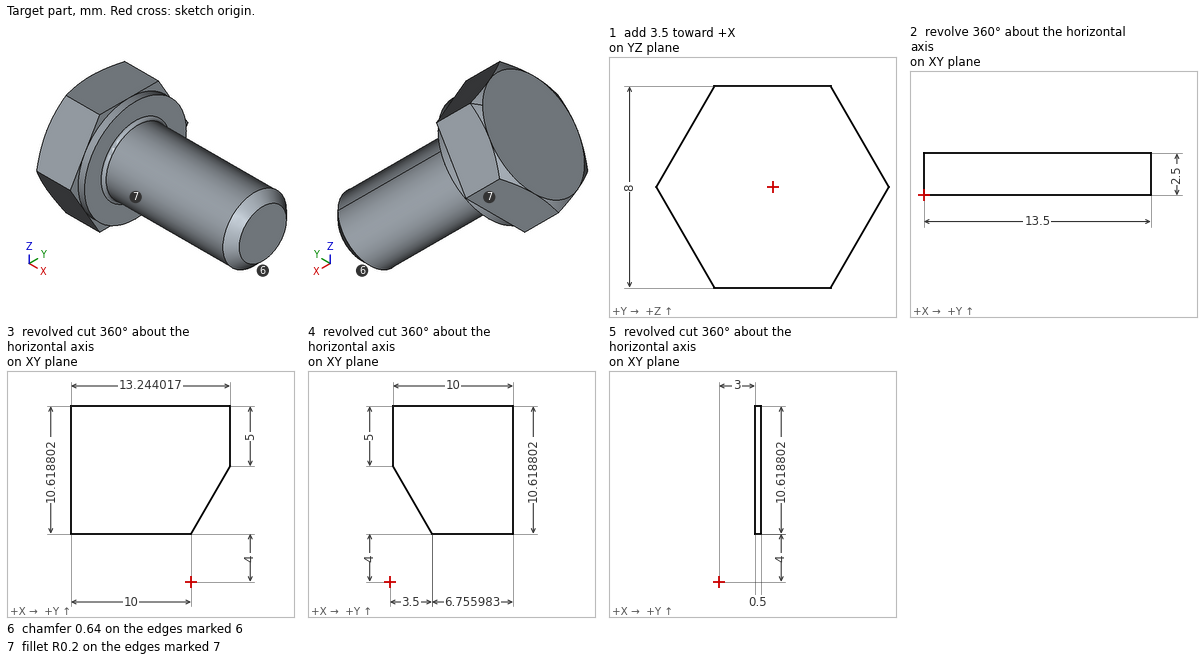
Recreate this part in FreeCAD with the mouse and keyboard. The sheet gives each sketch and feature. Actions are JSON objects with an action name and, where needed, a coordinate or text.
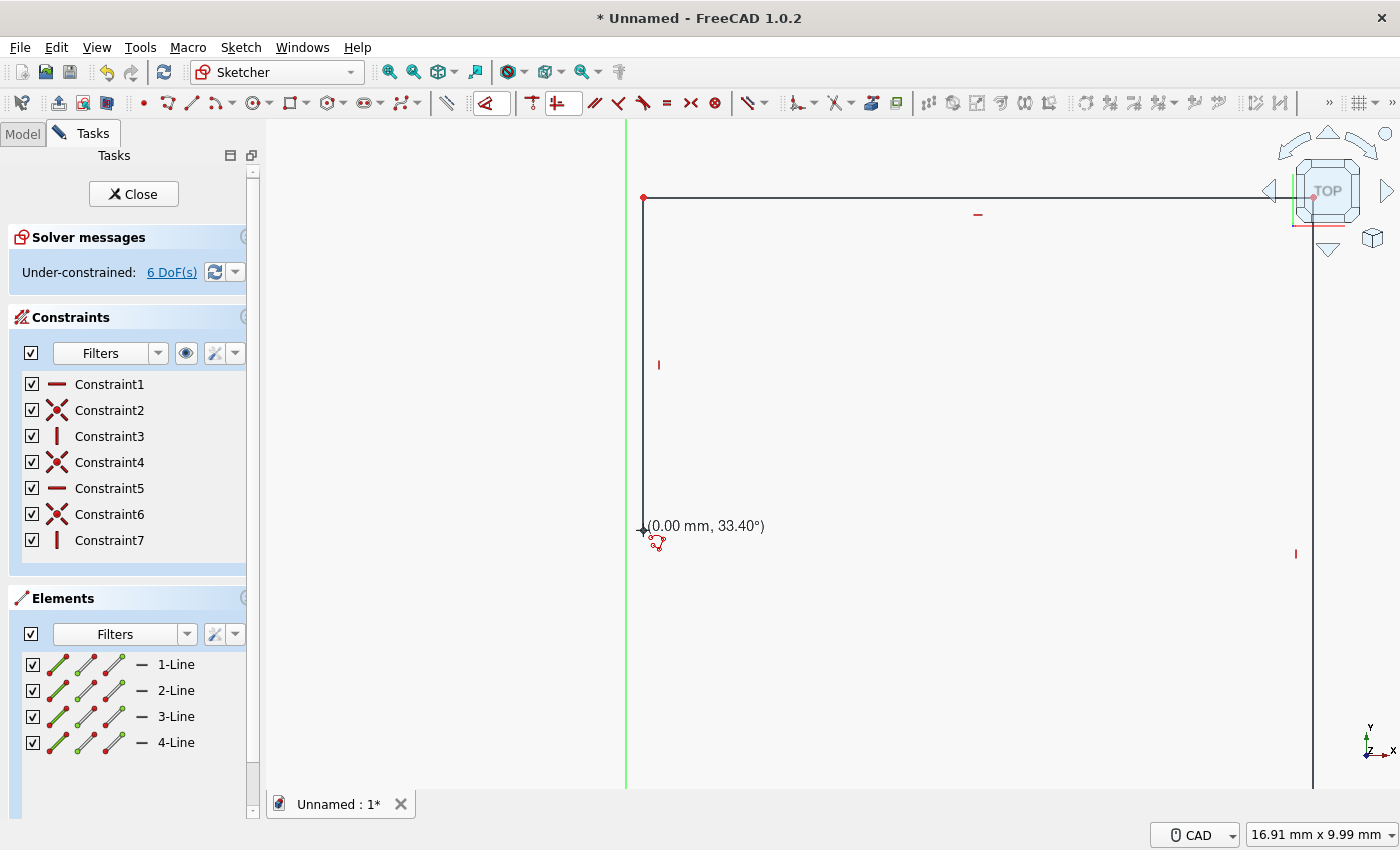
{"action": "scroll", "coordinate": [597, 266], "scroll_direction": "down", "scroll_amount": 4}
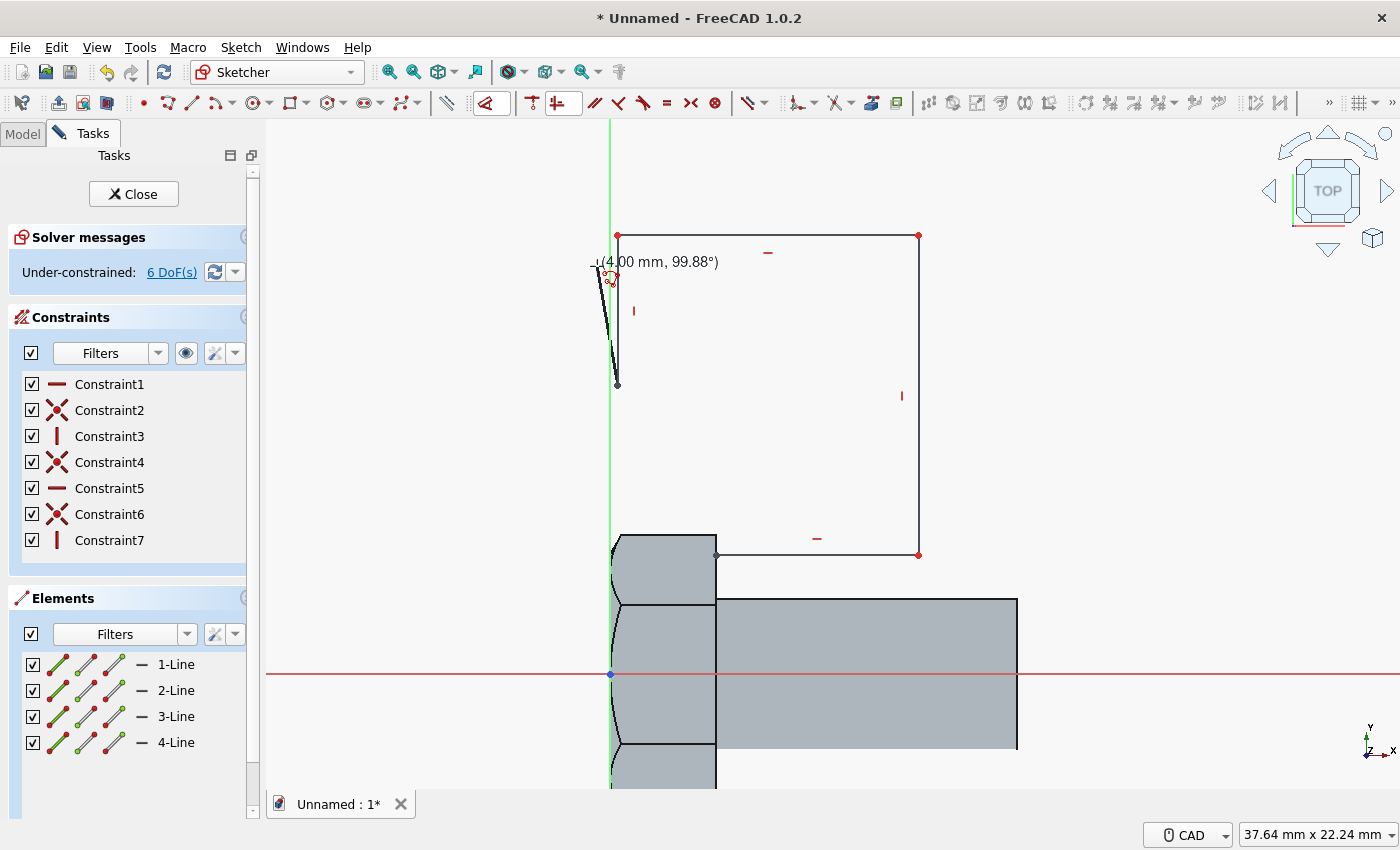
{"action": "left_click", "coordinate": [716, 555]}
{"action": "key", "text": "Escape"}
{"action": "key", "text": "Escape"}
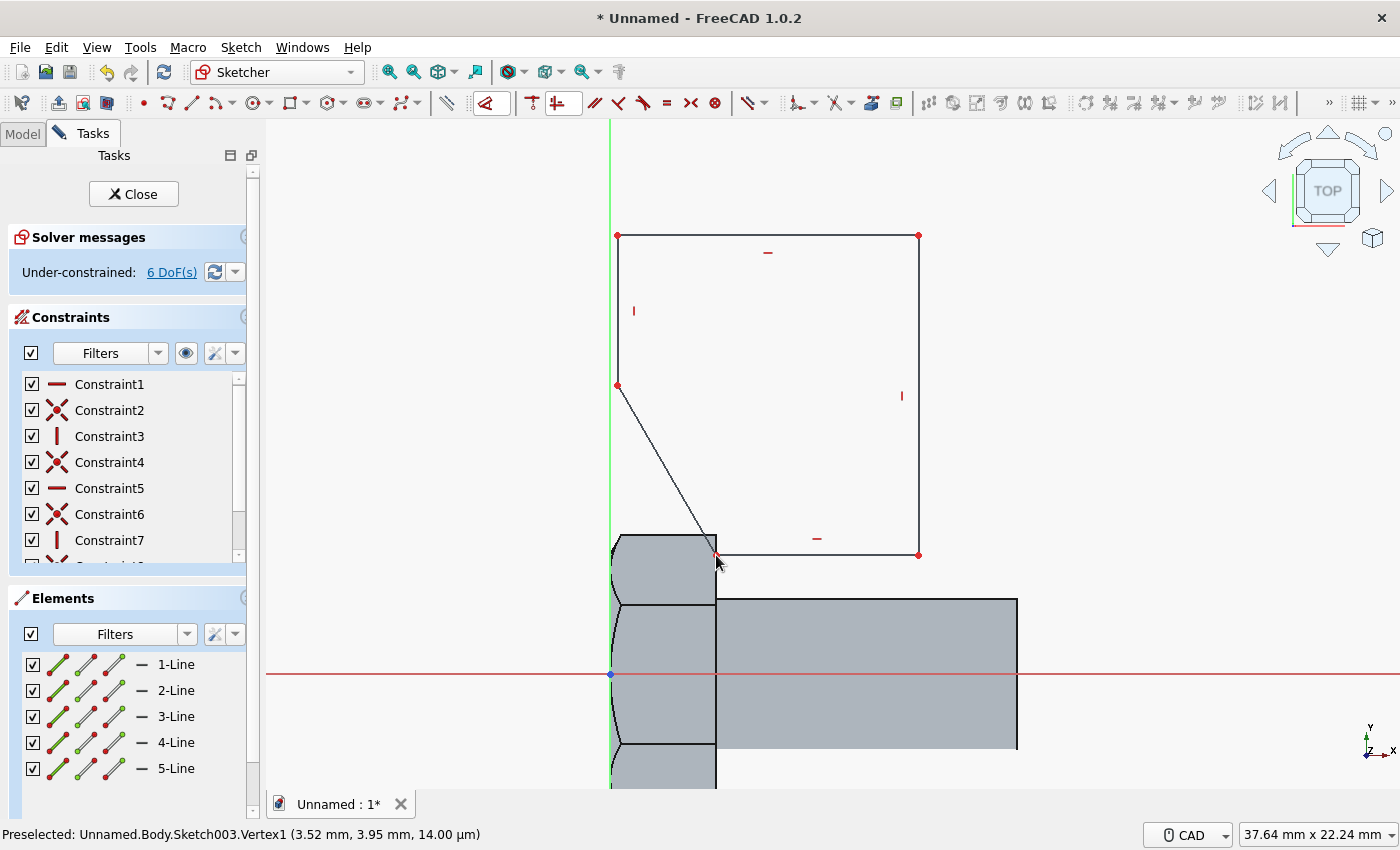
{"action": "scroll", "coordinate": [618, 280], "scroll_direction": "up", "scroll_amount": 4}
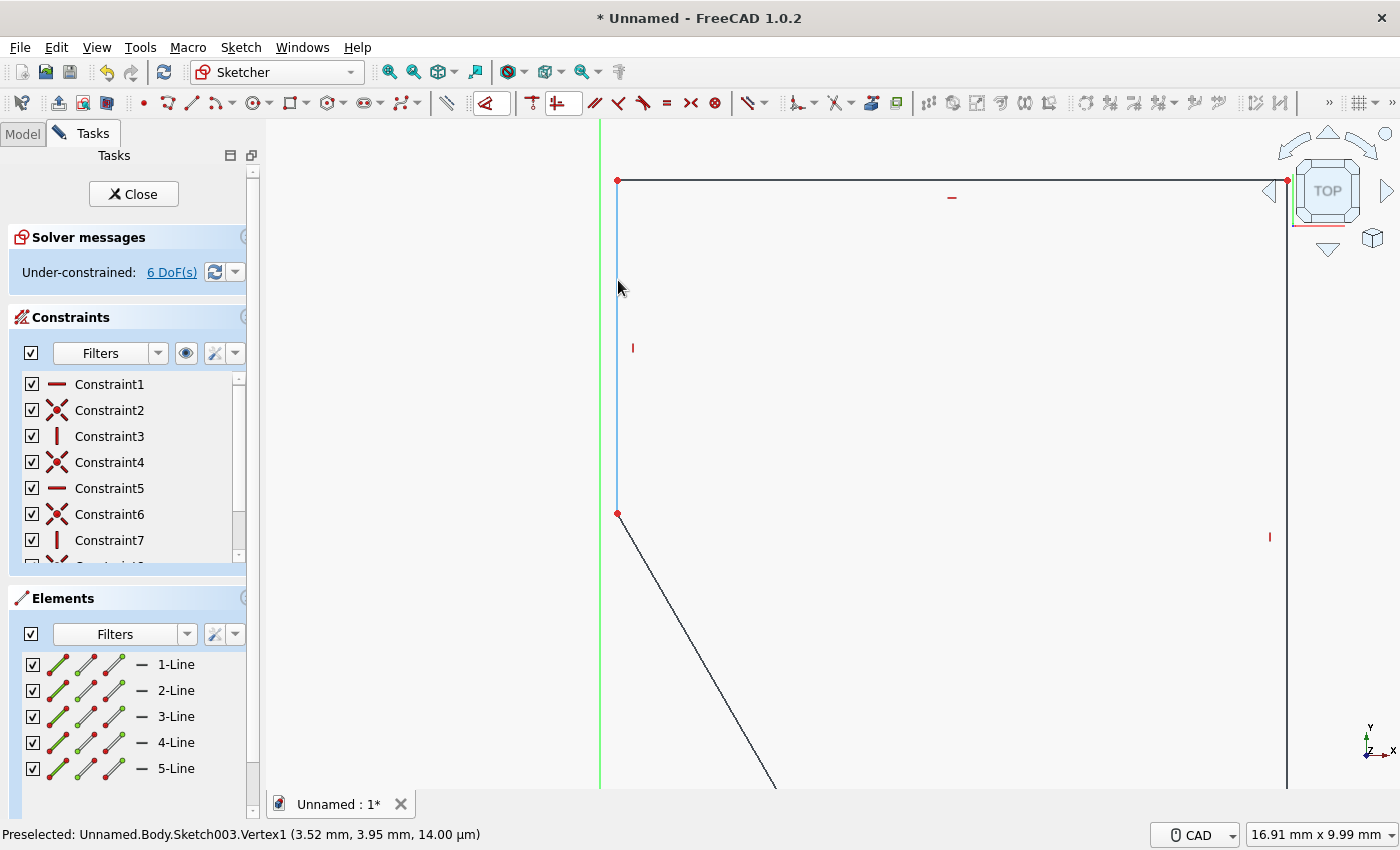
{"action": "left_click", "coordinate": [617, 280]}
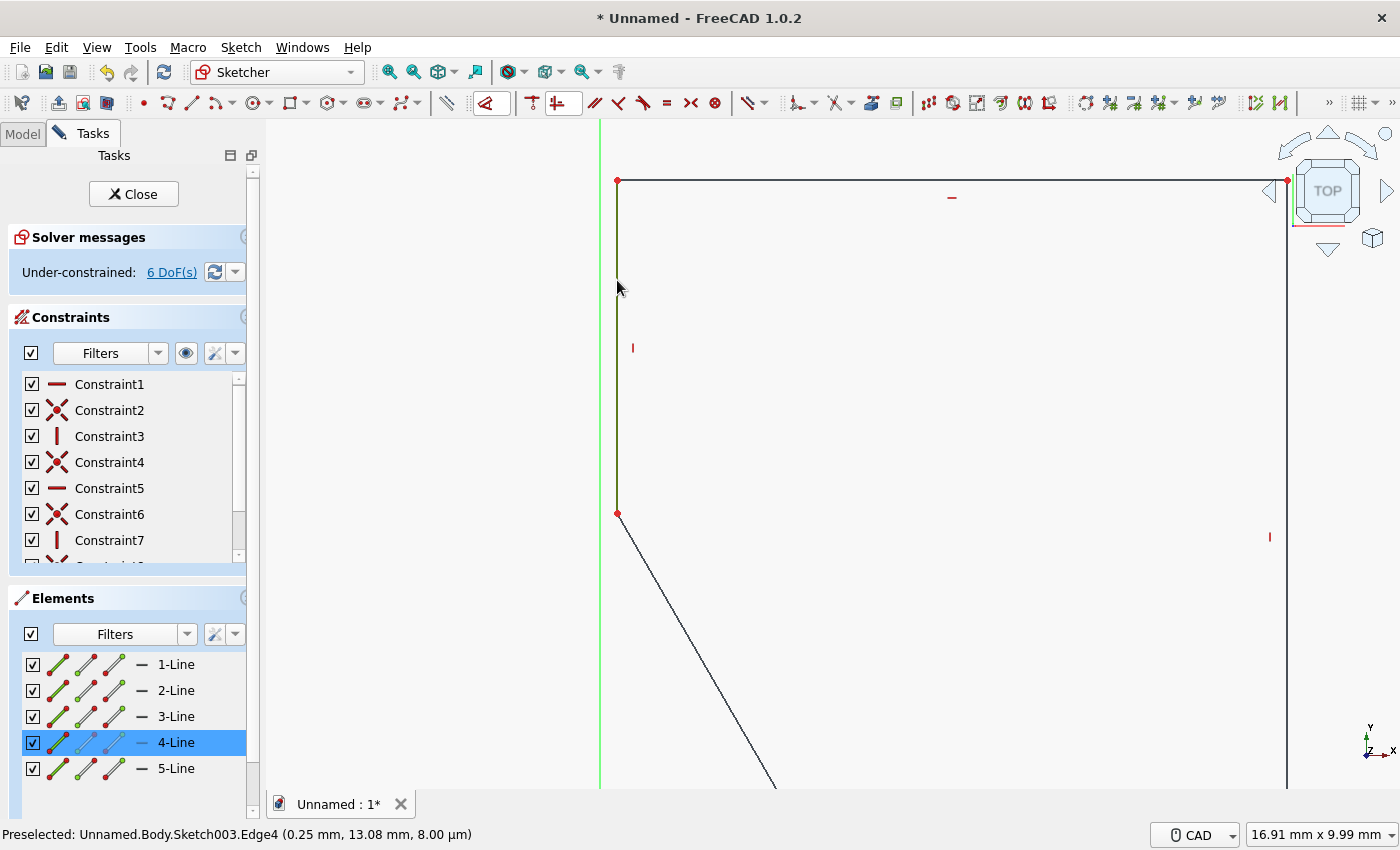
{"action": "key", "text": "i"}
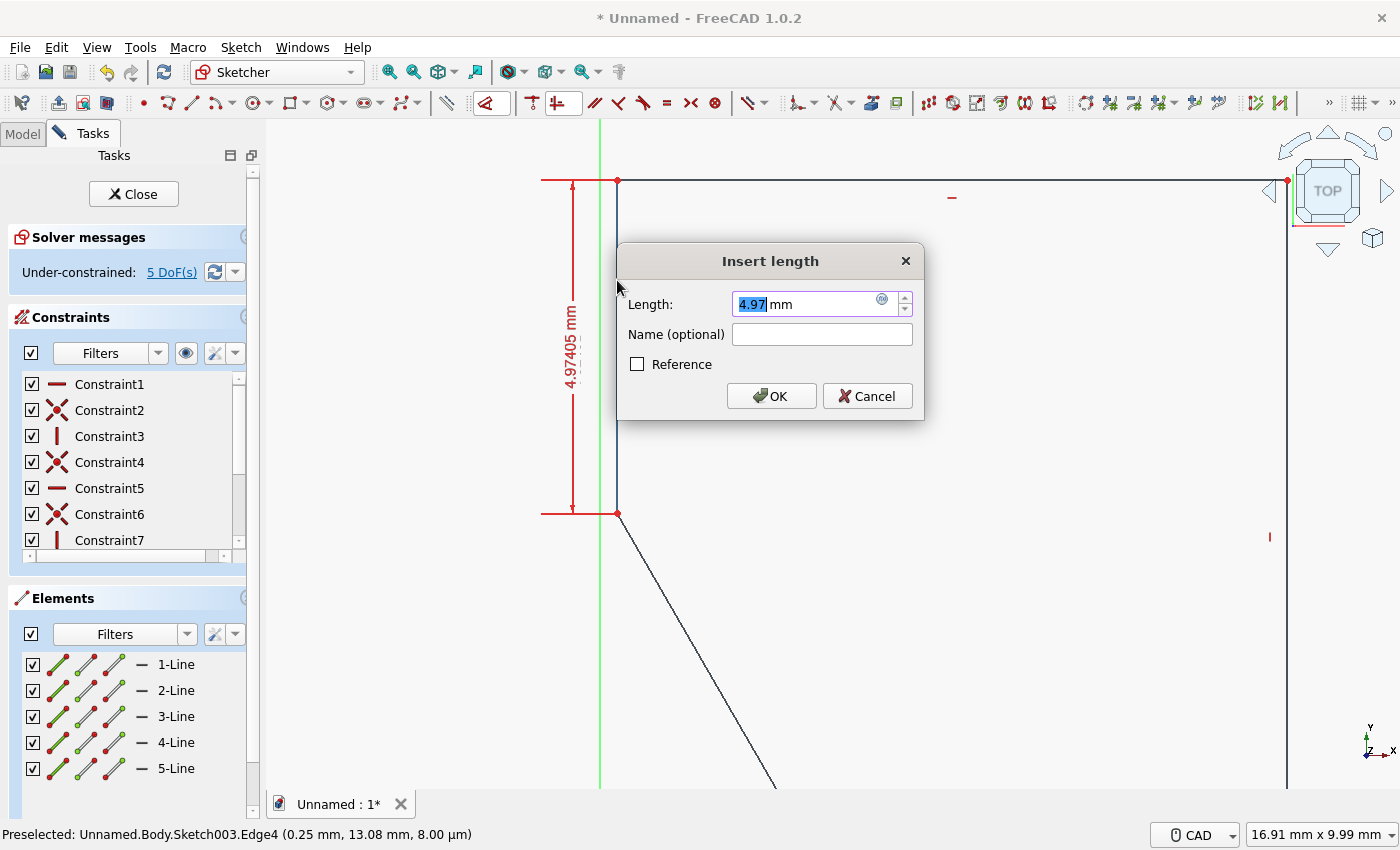
{"action": "type", "text": "5"}
{"action": "key", "text": "Return"}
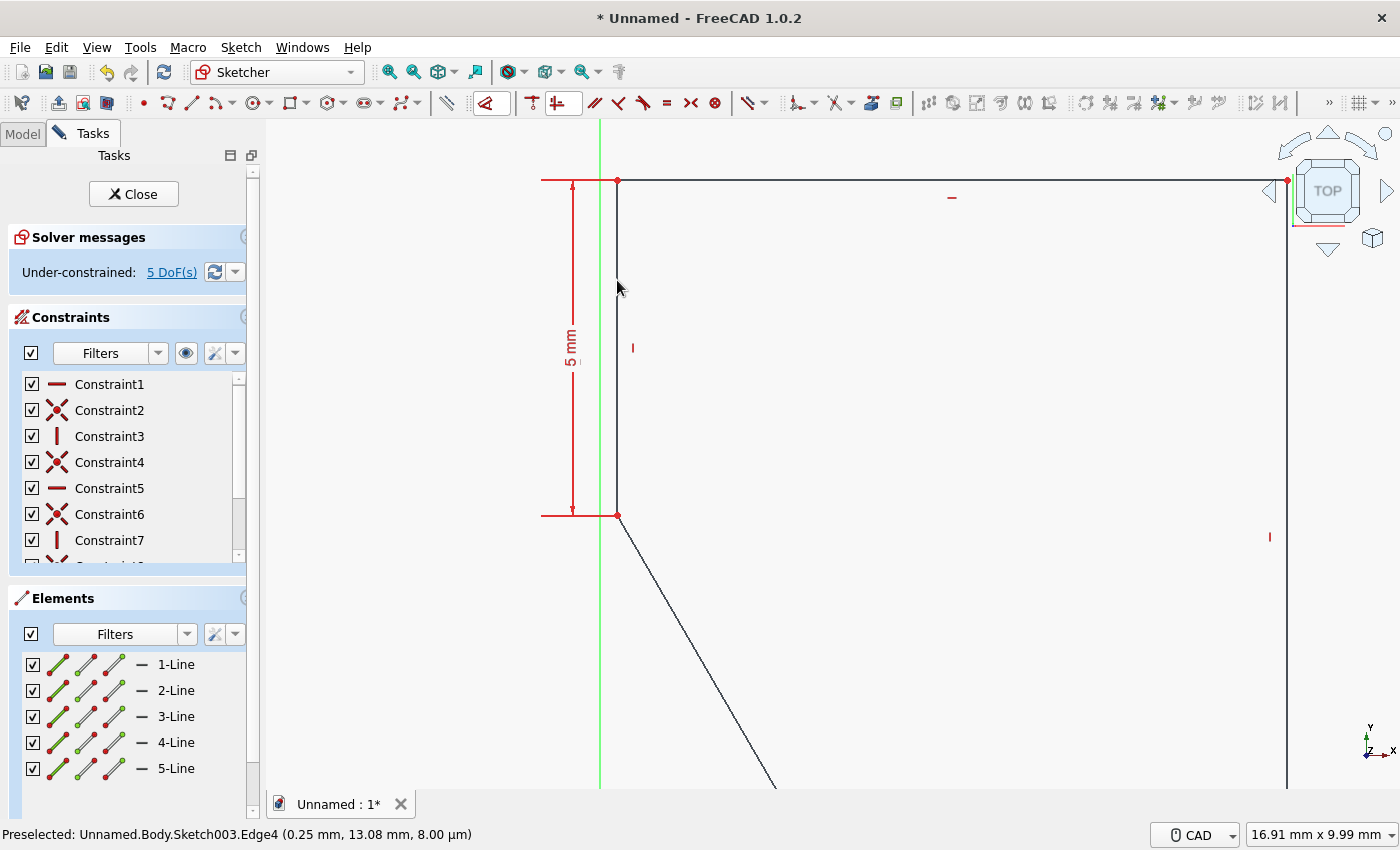
{"action": "left_click", "coordinate": [1086, 180]}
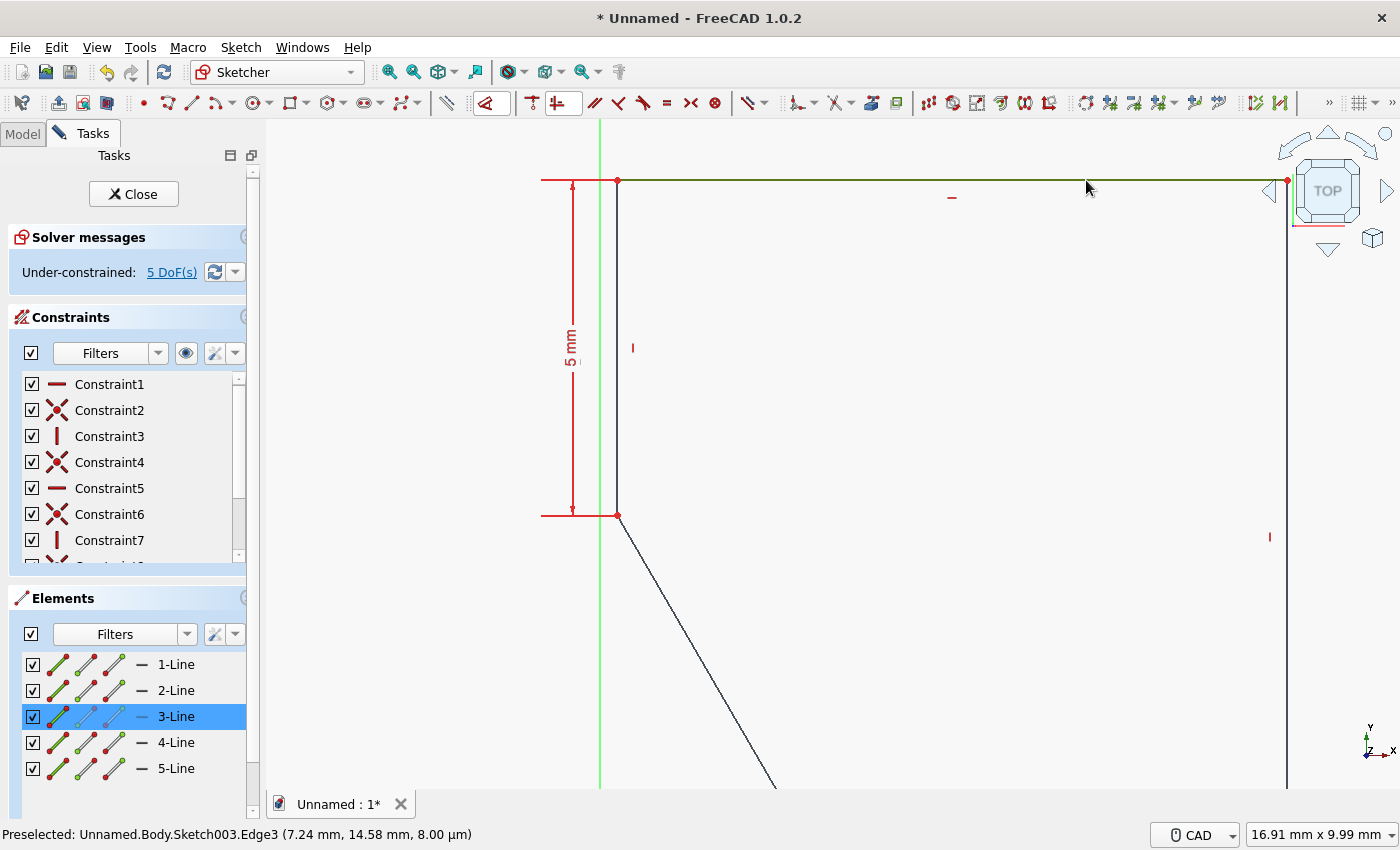
{"action": "left_click", "coordinate": [504, 104]}